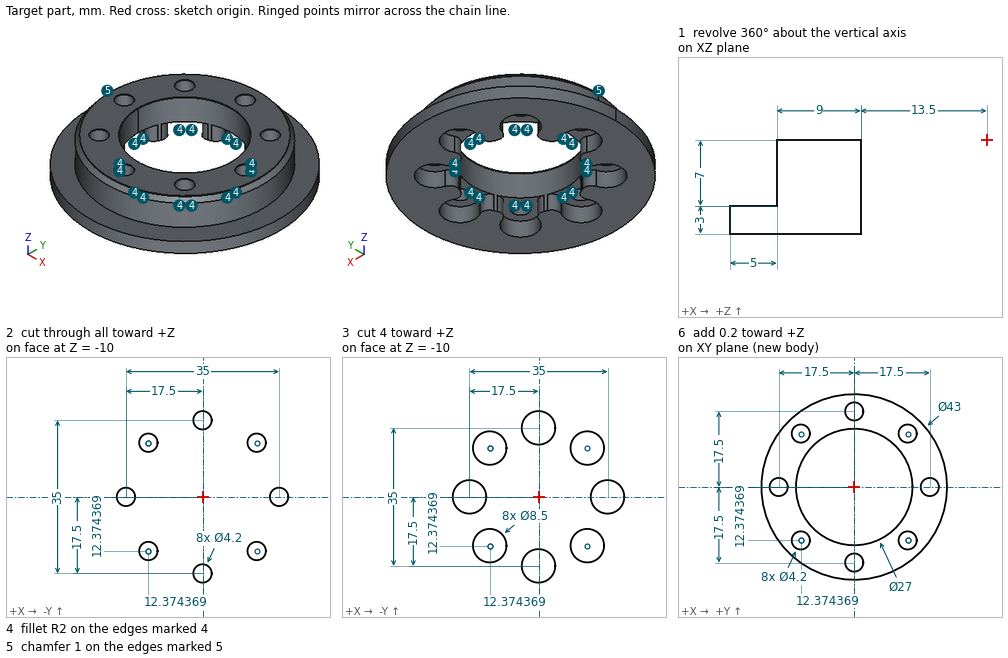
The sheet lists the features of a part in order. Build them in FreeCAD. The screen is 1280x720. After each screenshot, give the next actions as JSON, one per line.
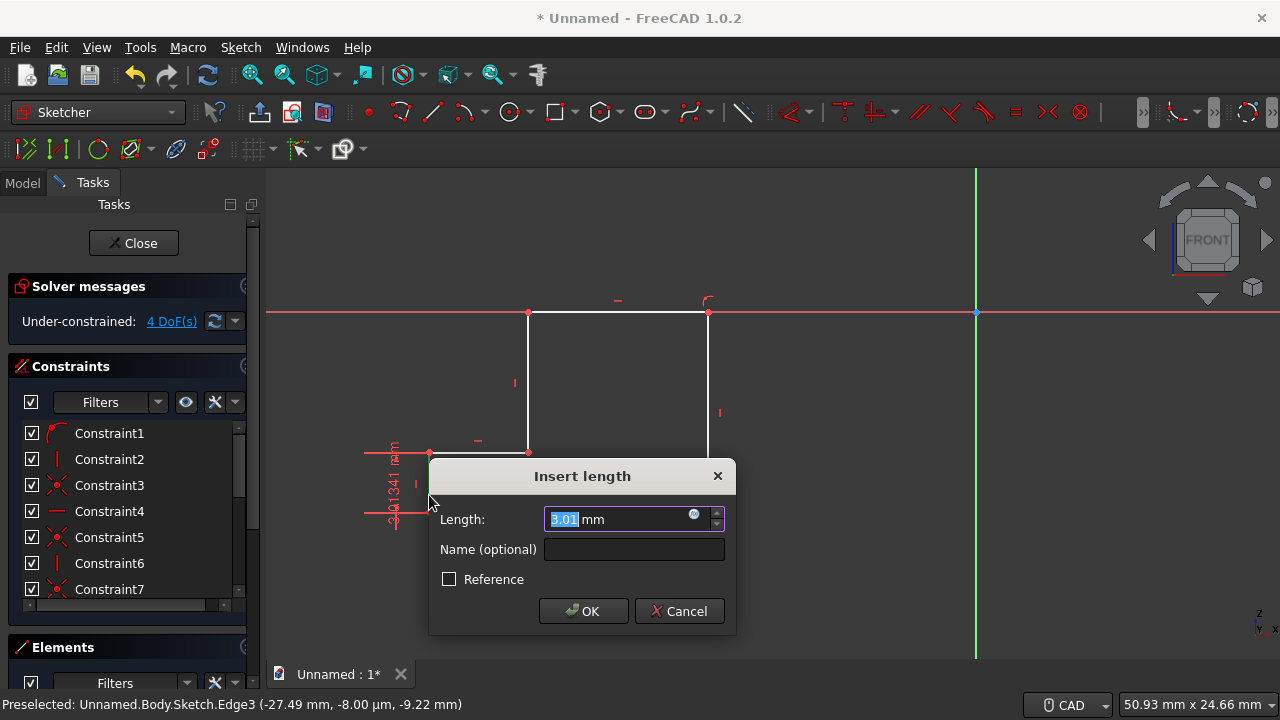
{"action": "type", "text": "3"}
{"action": "key", "text": "Return"}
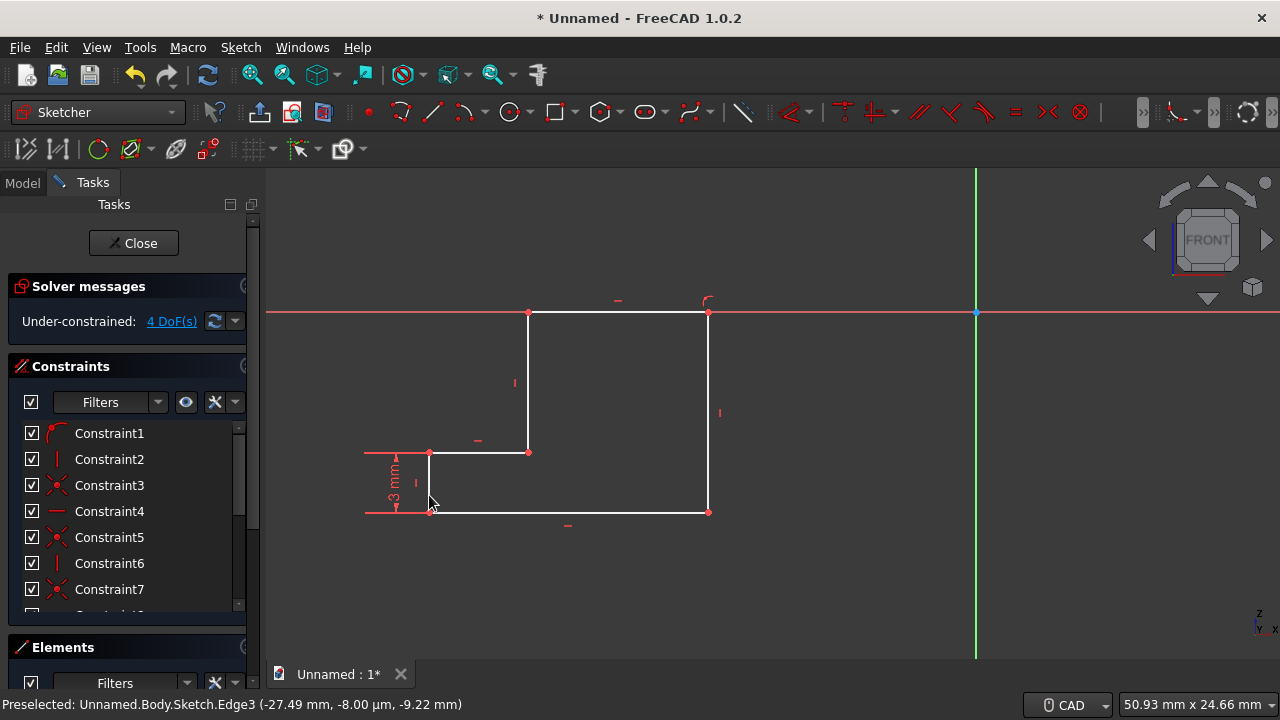
{"action": "left_click", "coordinate": [459, 453]}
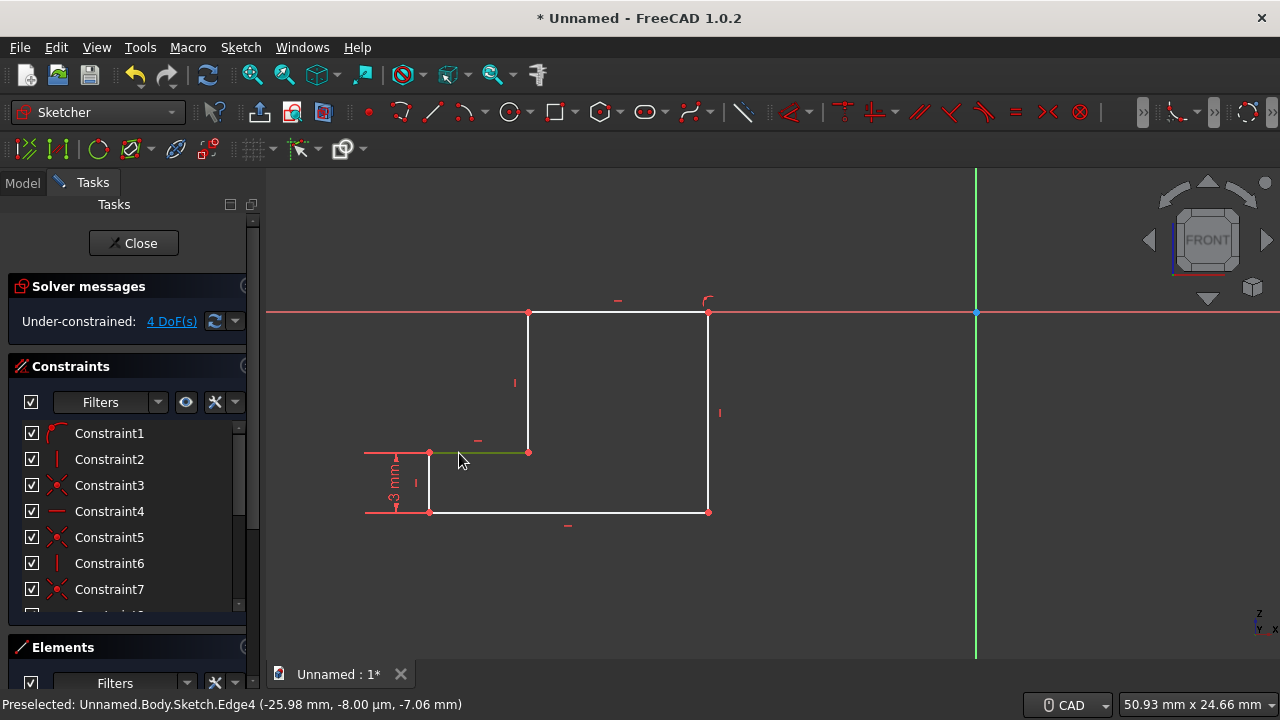
{"action": "key", "text": "l"}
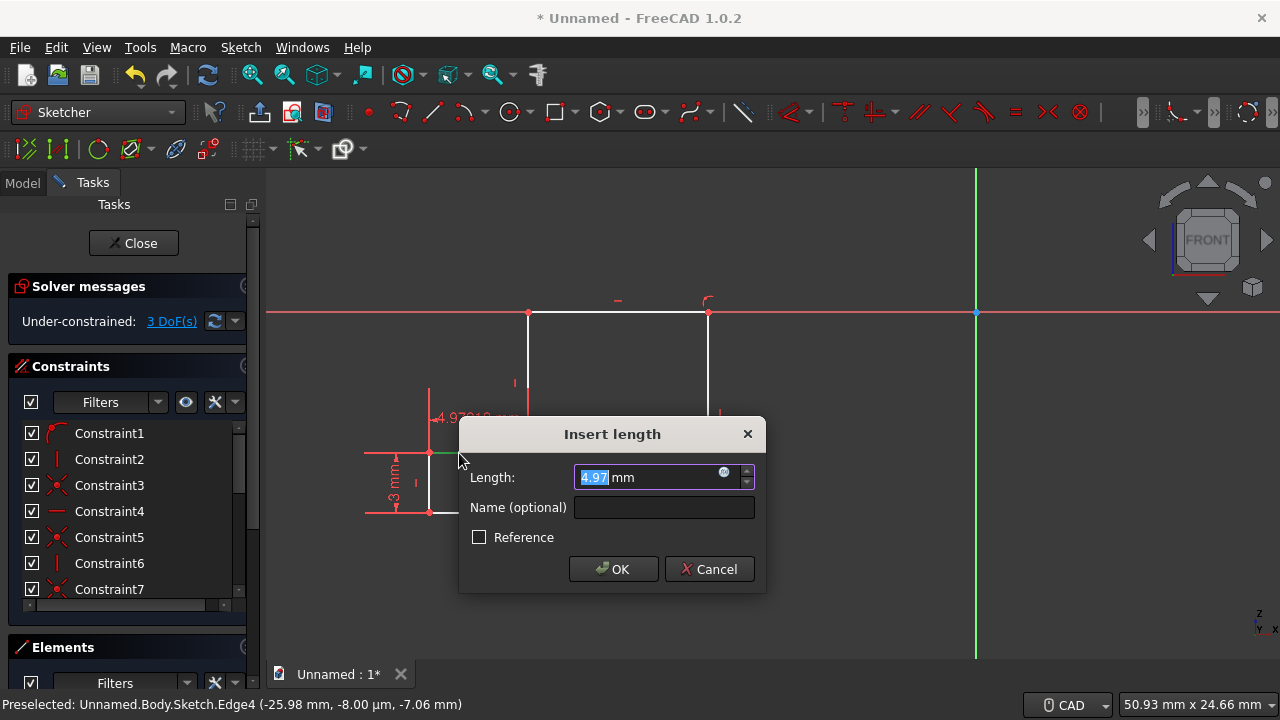
{"action": "type", "text": "5"}
{"action": "key", "text": "Return"}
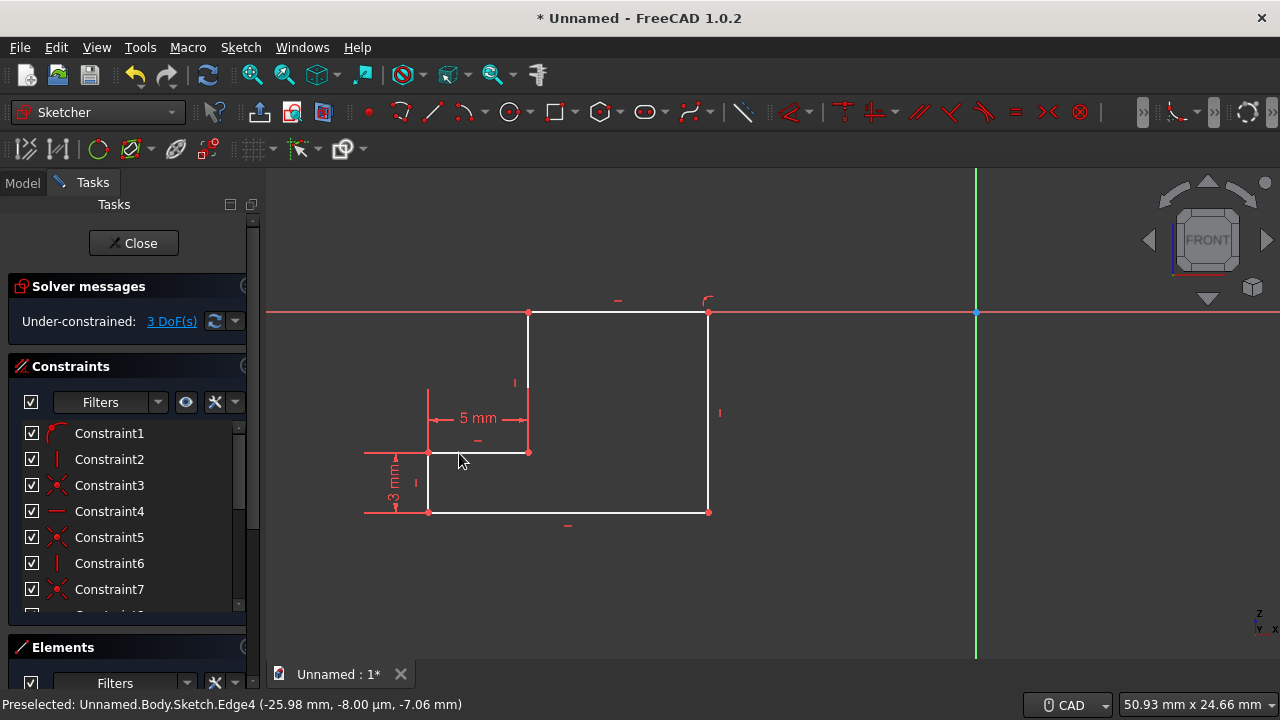
{"action": "left_click", "coordinate": [528, 411]}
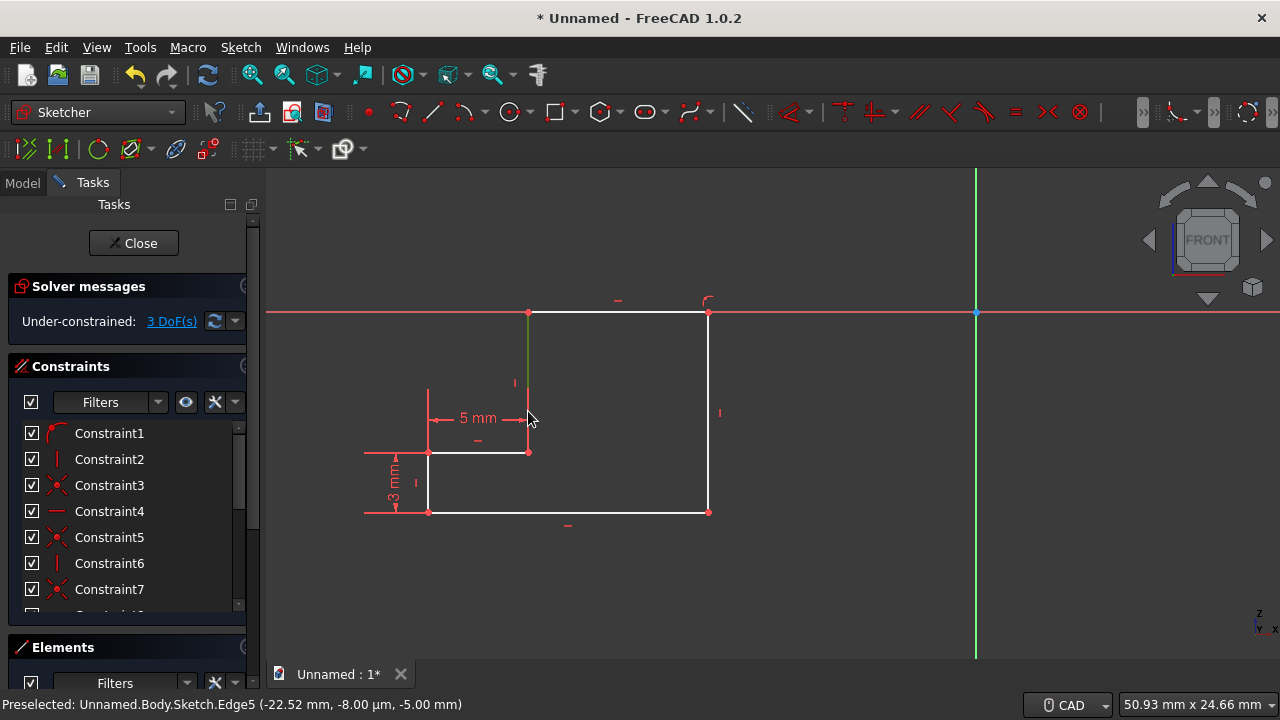
{"action": "left_click", "coordinate": [812, 112]}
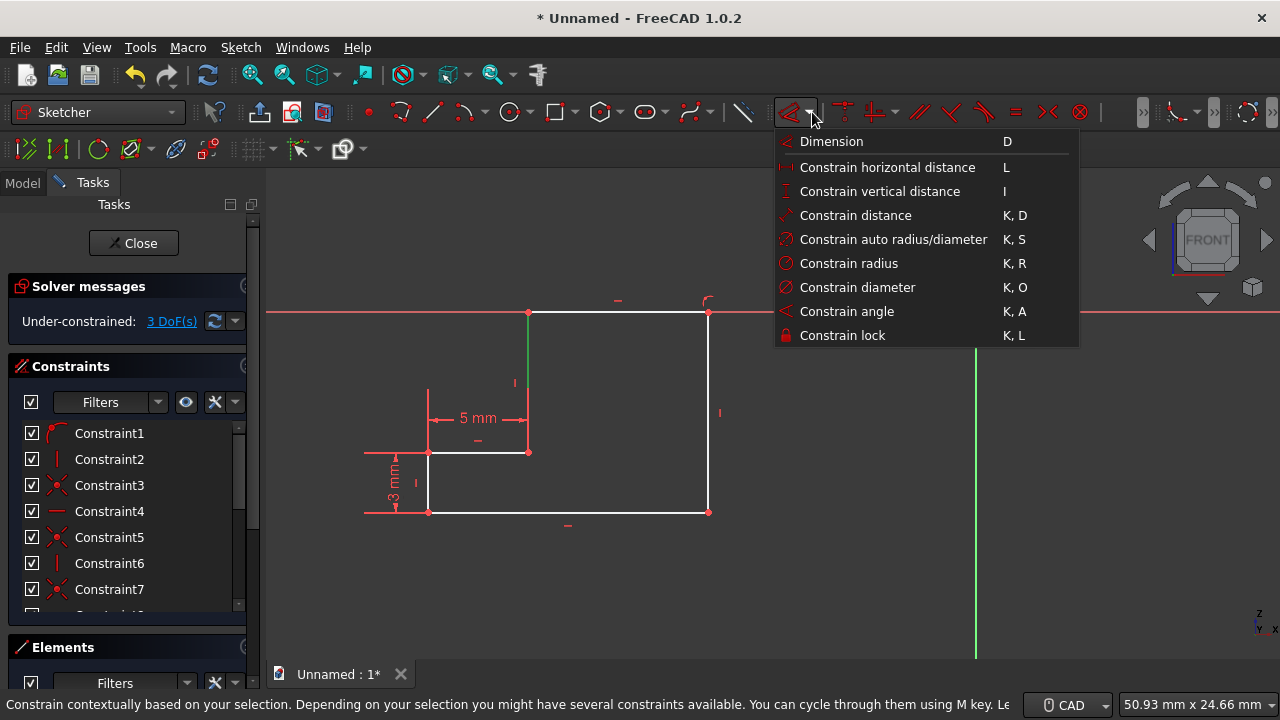
{"action": "left_click", "coordinate": [927, 191]}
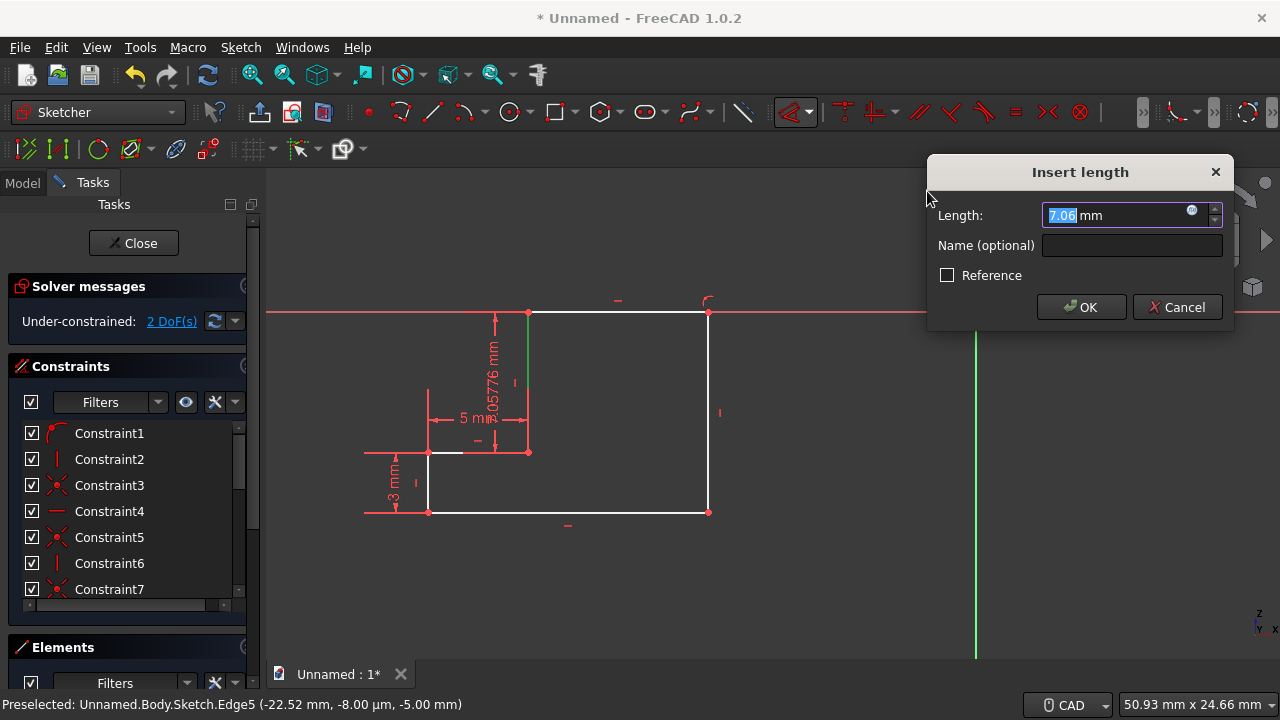
{"action": "type", "text": "7"}
{"action": "key", "text": "Return"}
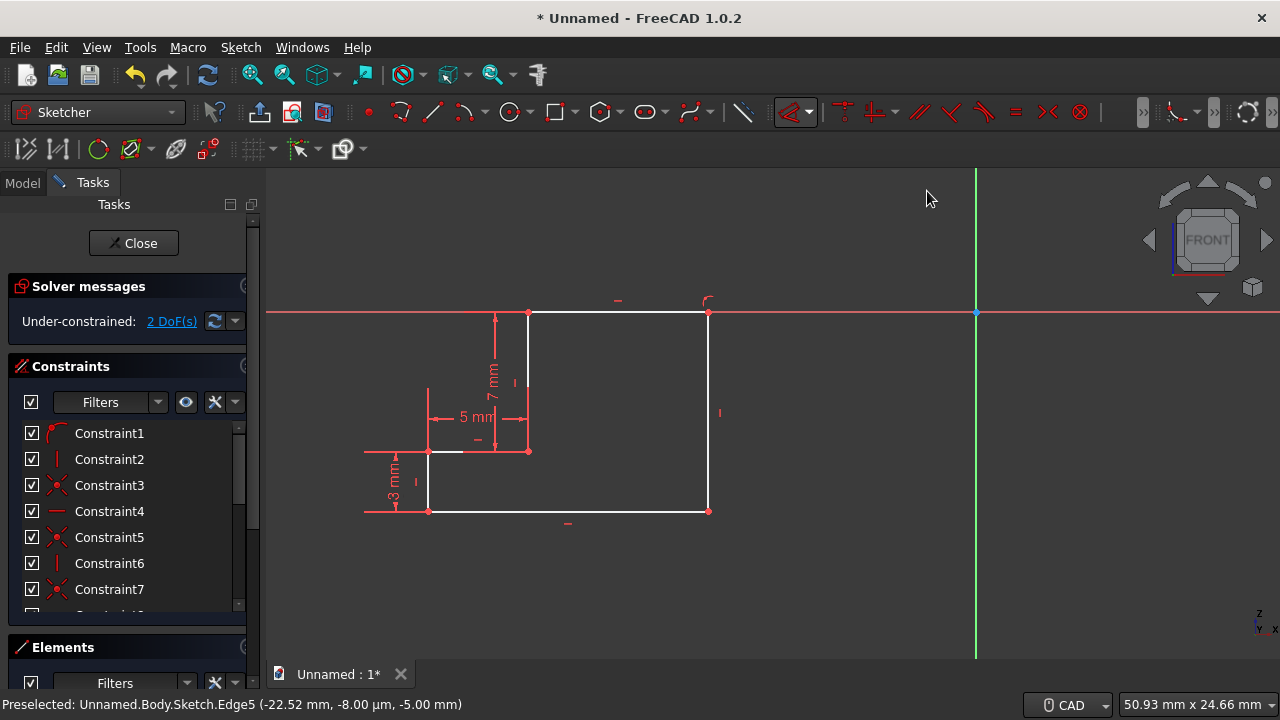
{"action": "left_click", "coordinate": [582, 312]}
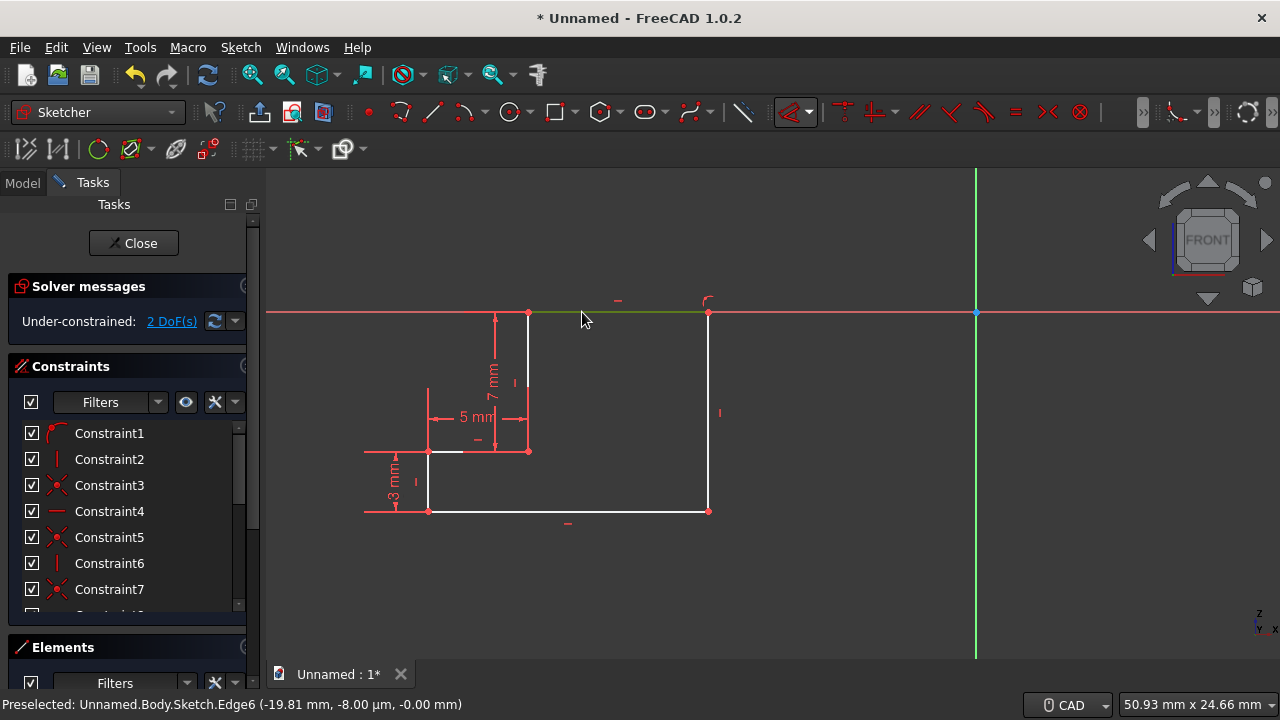
{"action": "key", "text": "l"}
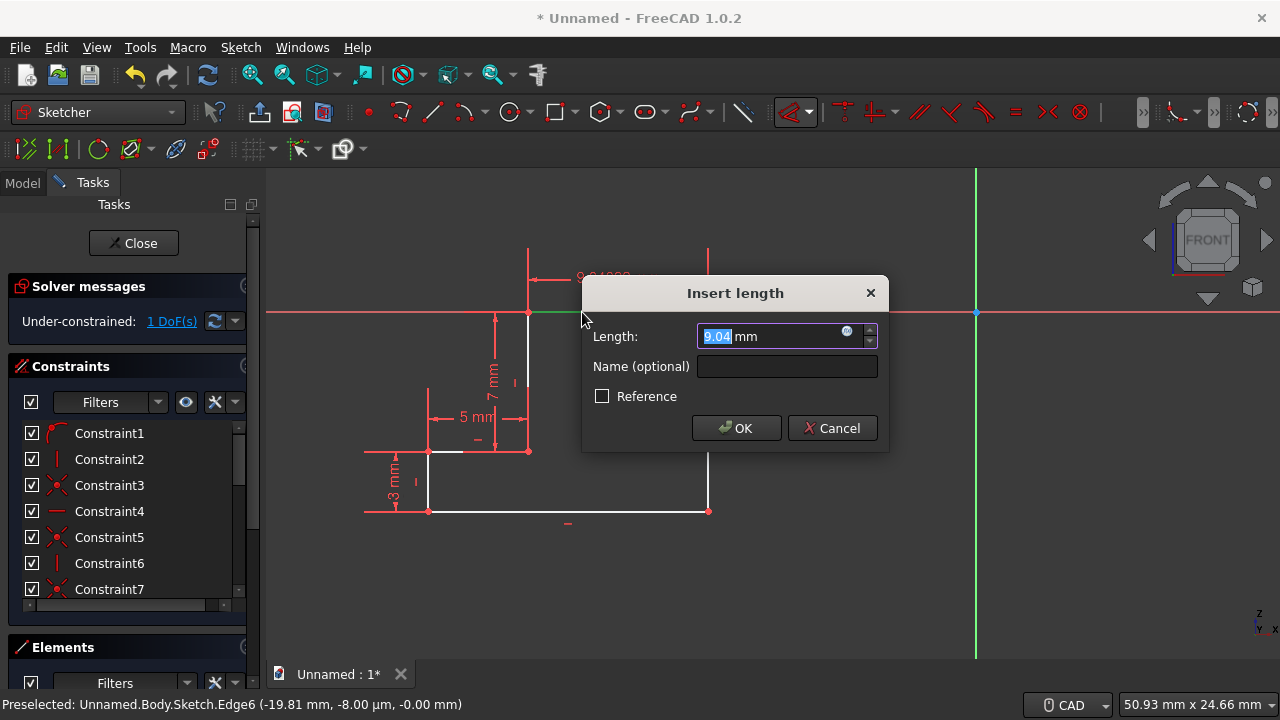
{"action": "type", "text": "9"}
{"action": "key", "text": "Return"}